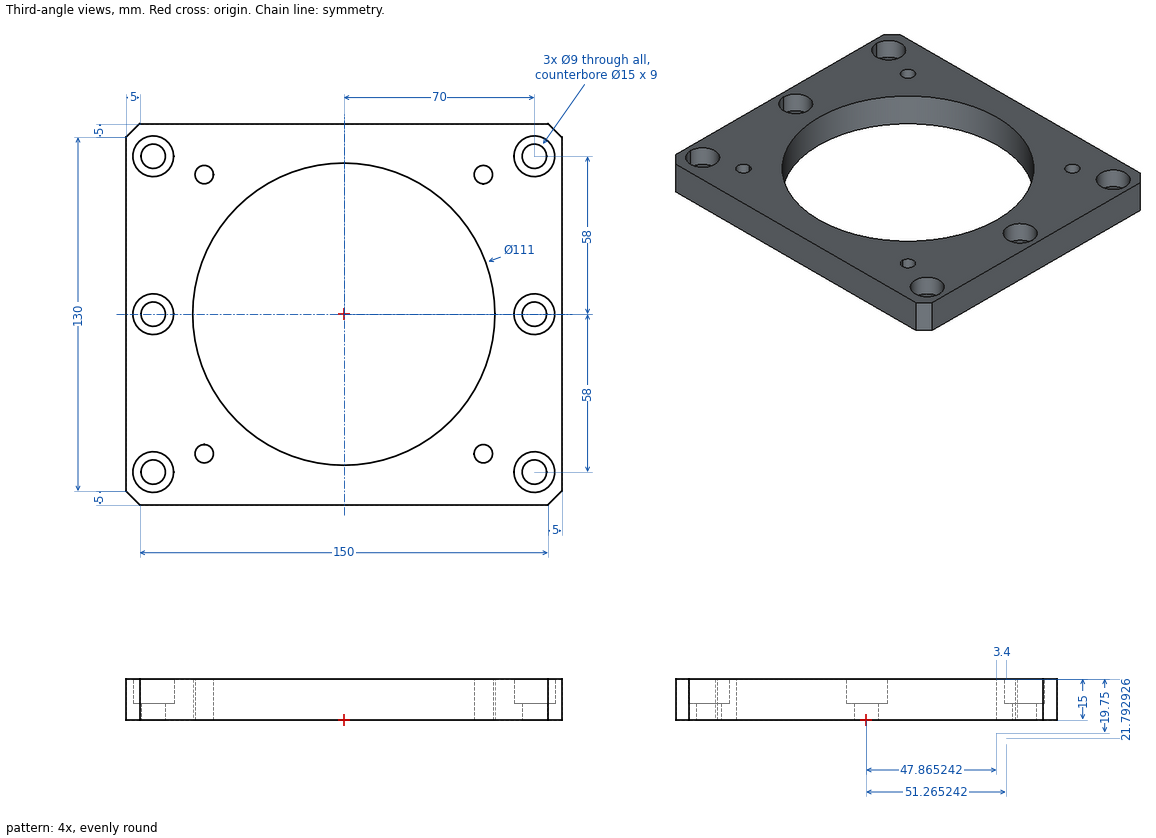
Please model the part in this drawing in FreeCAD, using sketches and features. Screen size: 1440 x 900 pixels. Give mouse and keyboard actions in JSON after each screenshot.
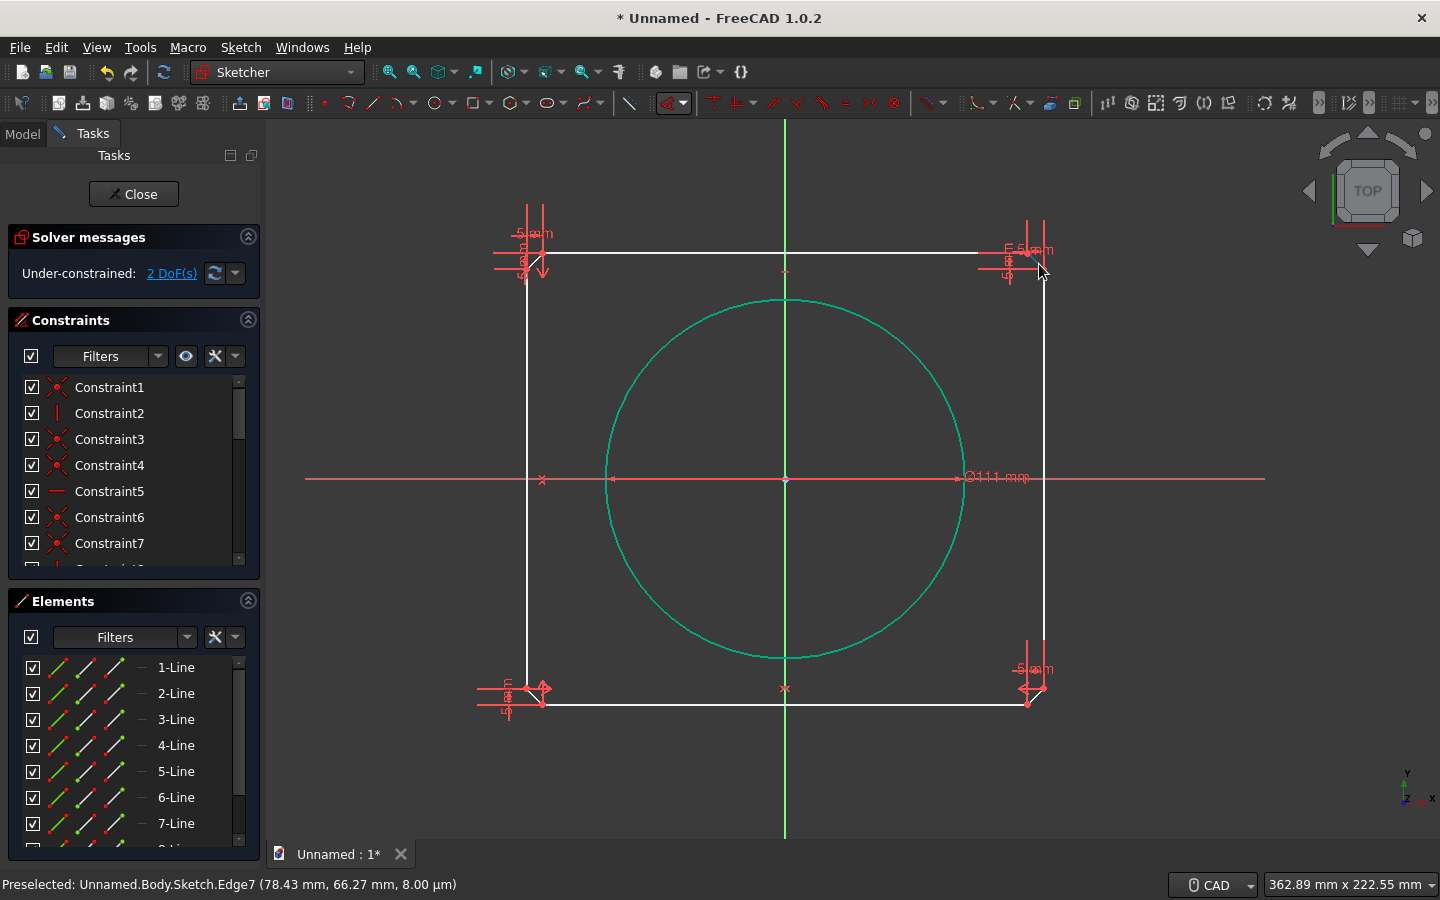
{"action": "left_click", "coordinate": [527, 395]}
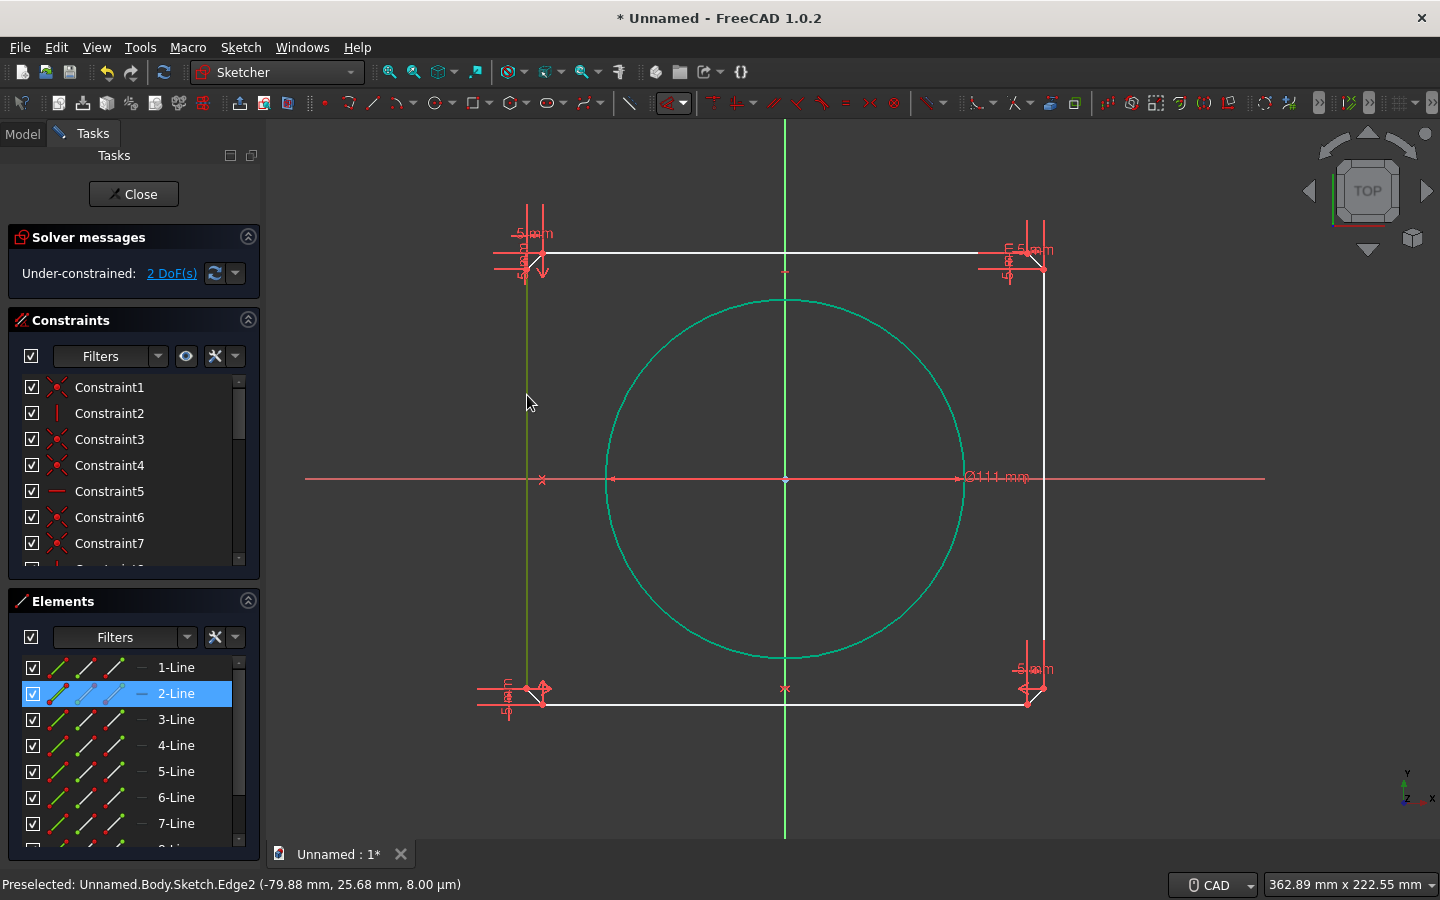
{"action": "left_click", "coordinate": [686, 104]}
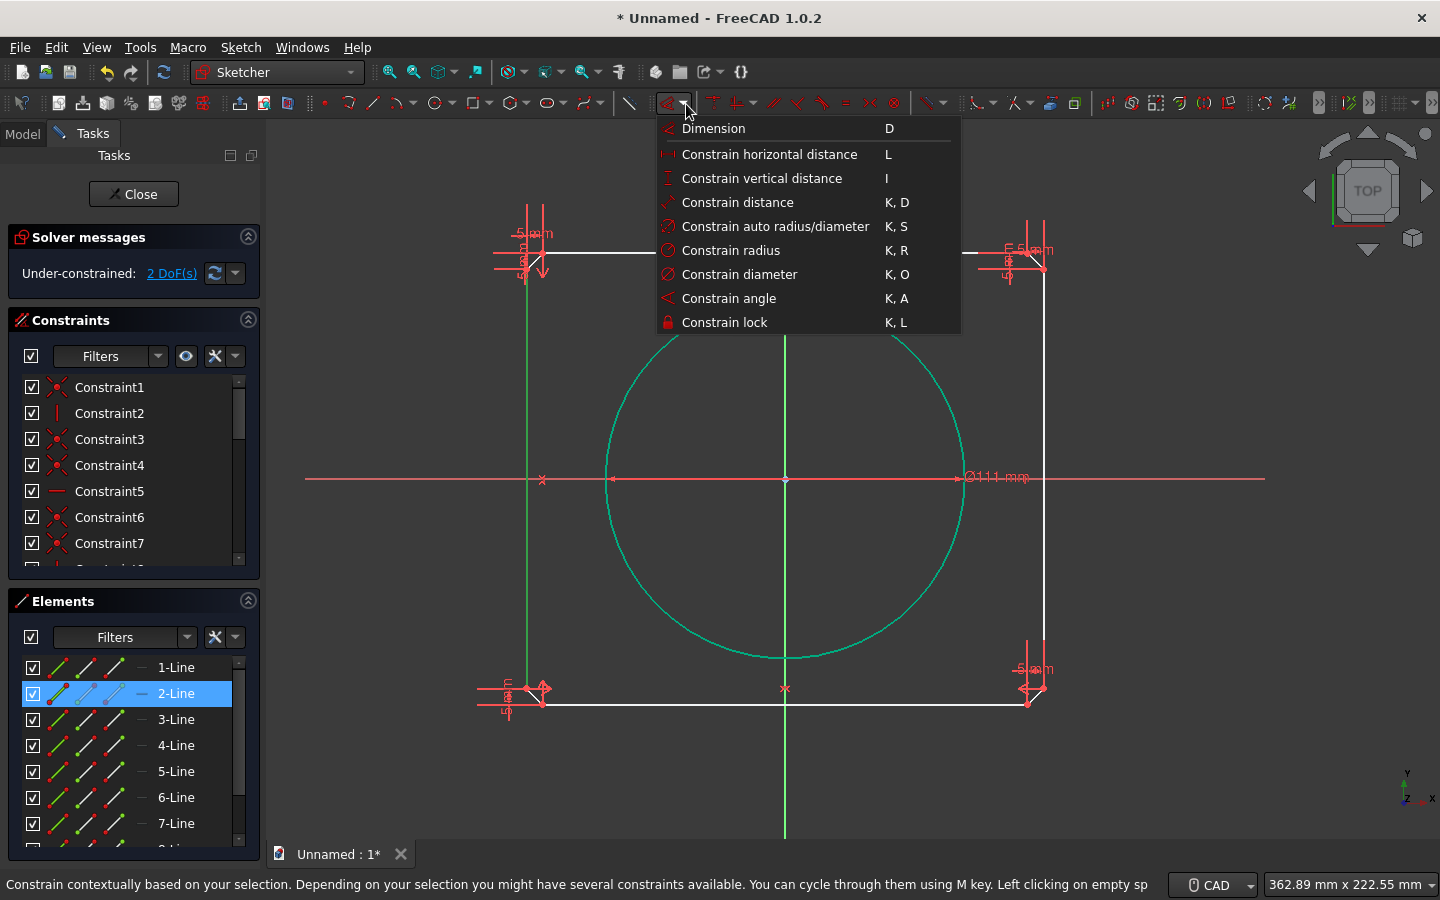
{"action": "left_click", "coordinate": [809, 178]}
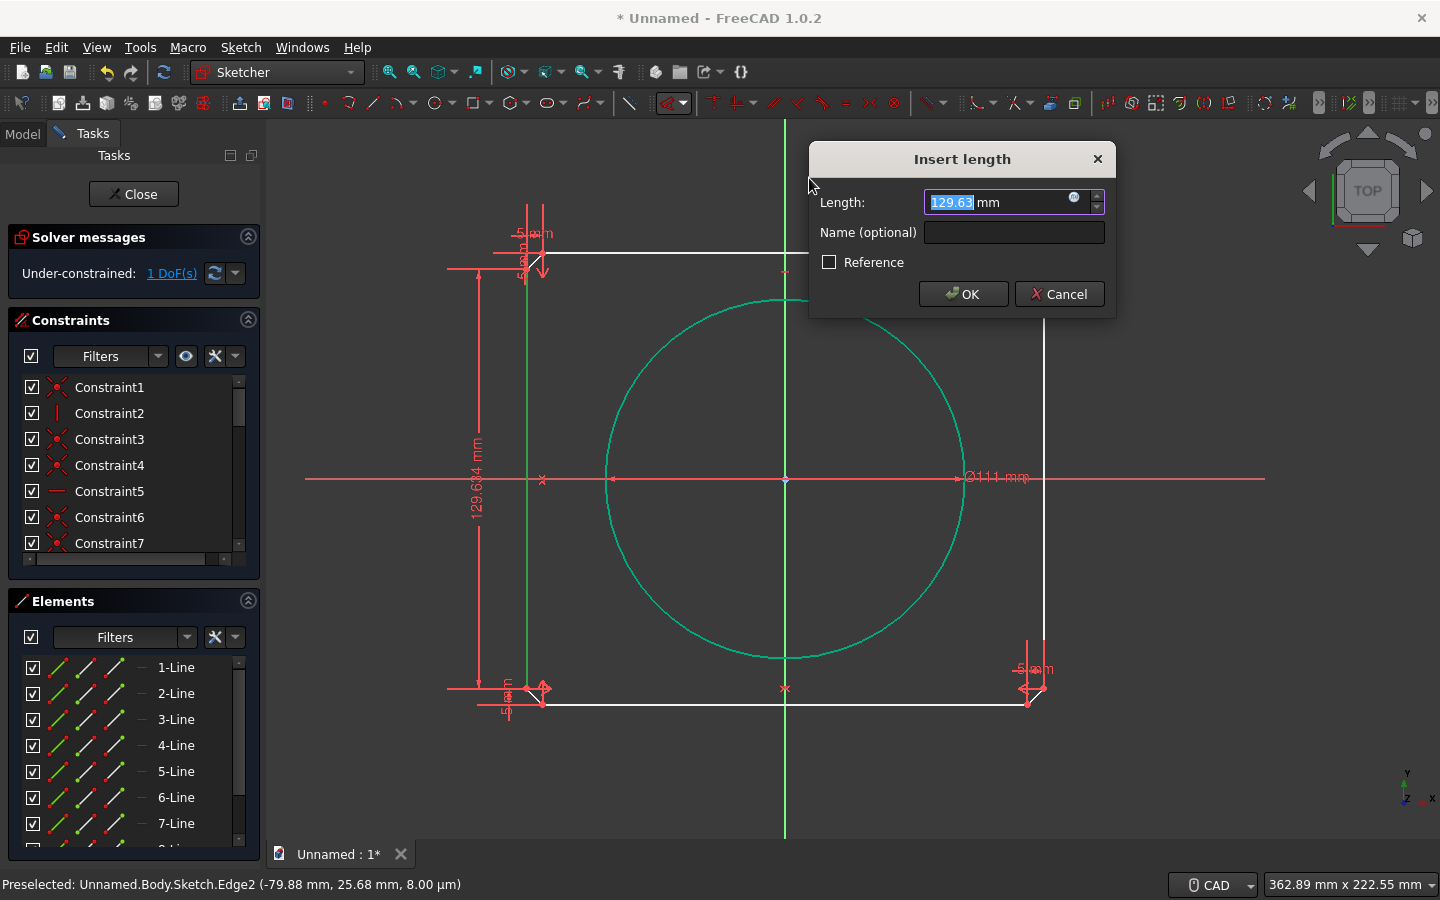
{"action": "type", "text": "130"}
{"action": "key", "text": "Return"}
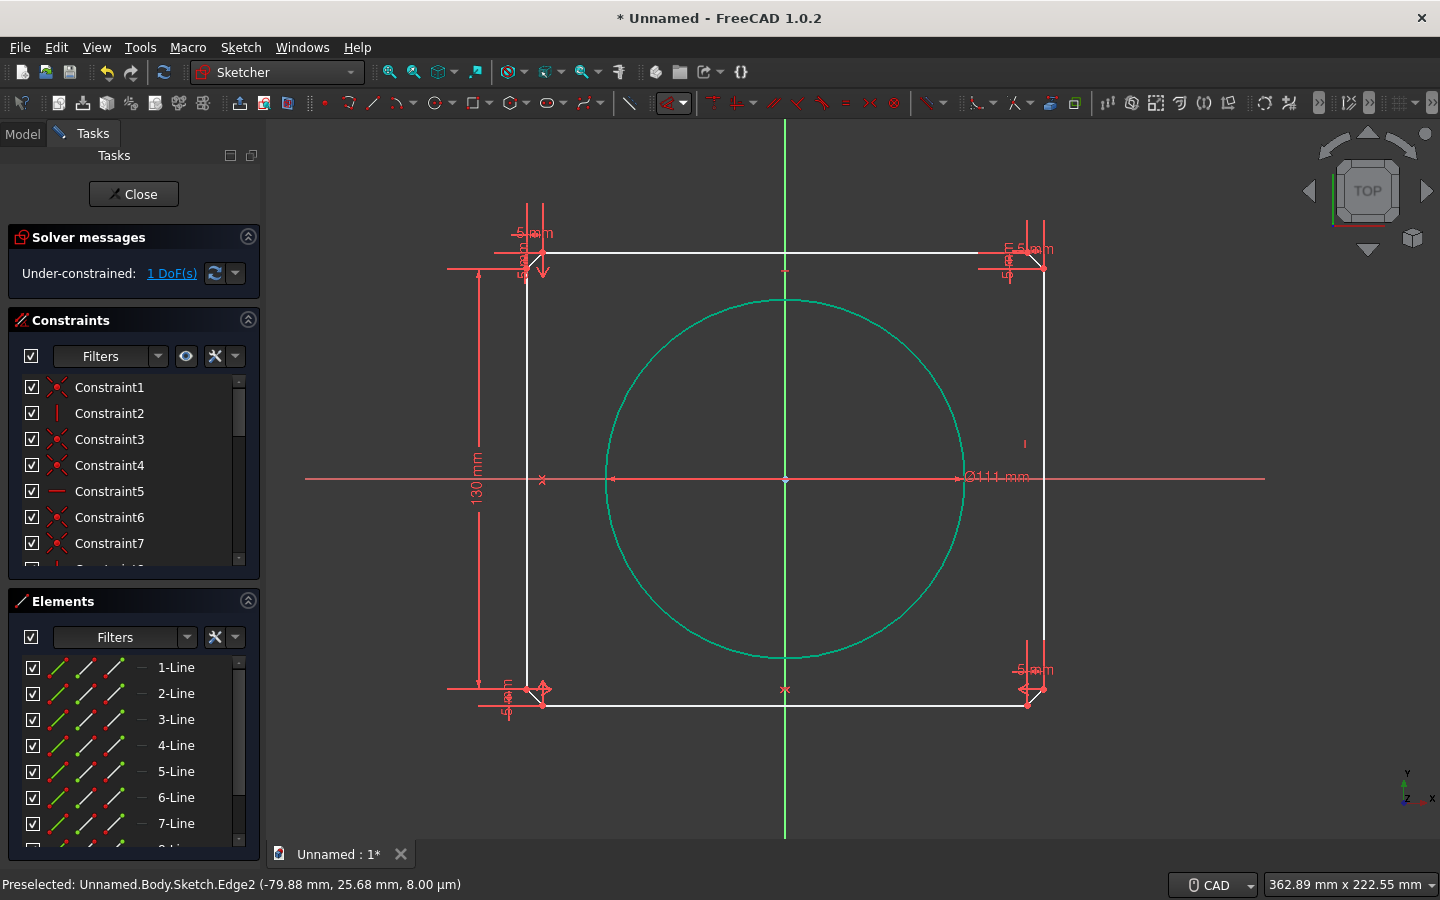
{"action": "left_click", "coordinate": [688, 706]}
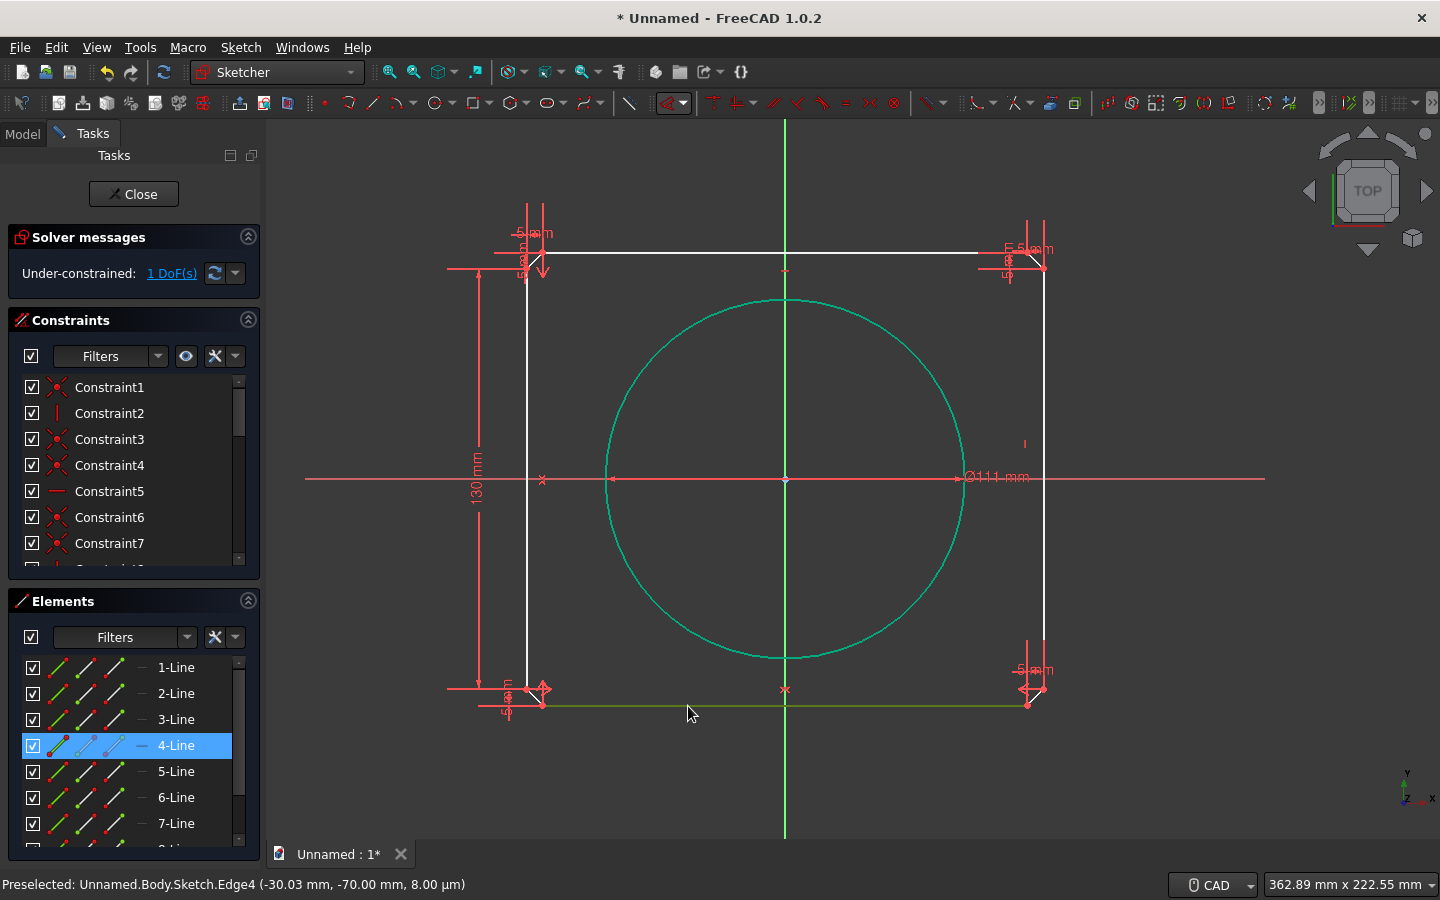
{"action": "left_click", "coordinate": [686, 104]}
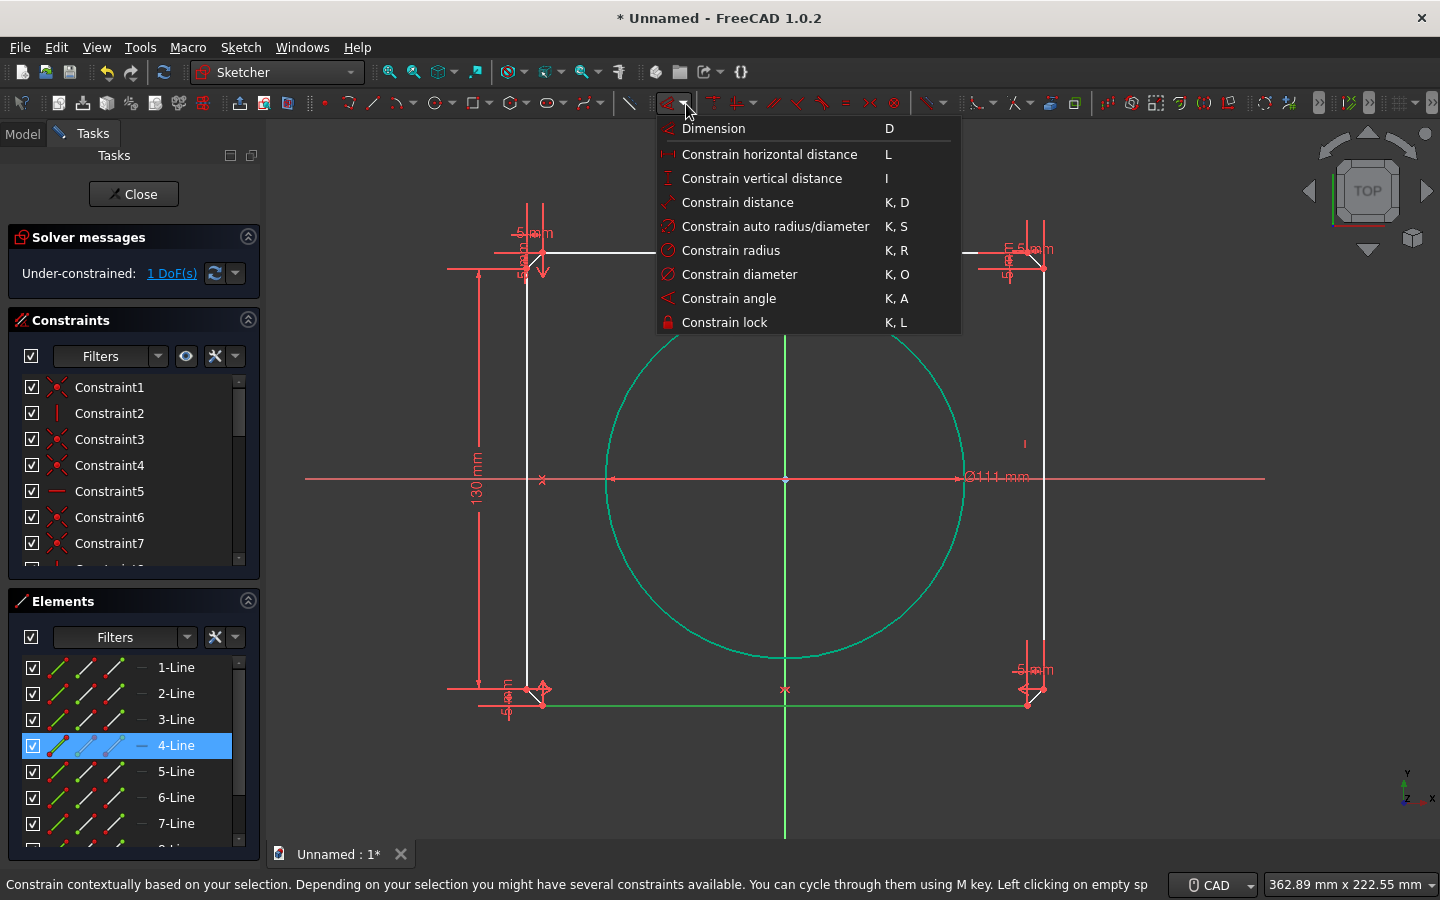
{"action": "left_click", "coordinate": [809, 154]}